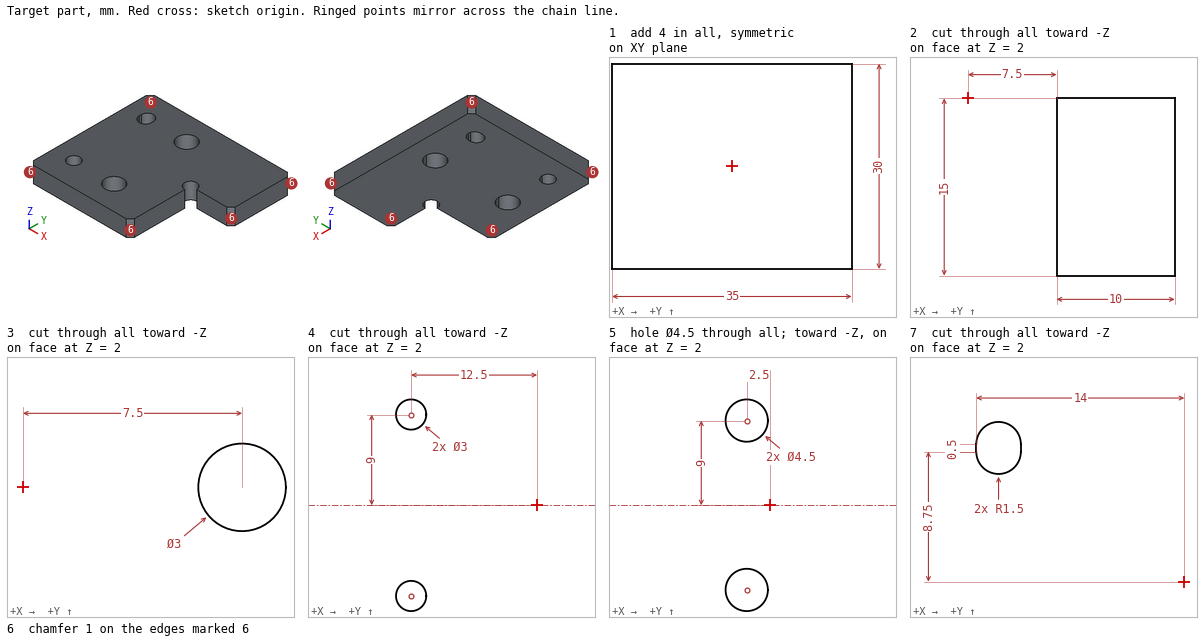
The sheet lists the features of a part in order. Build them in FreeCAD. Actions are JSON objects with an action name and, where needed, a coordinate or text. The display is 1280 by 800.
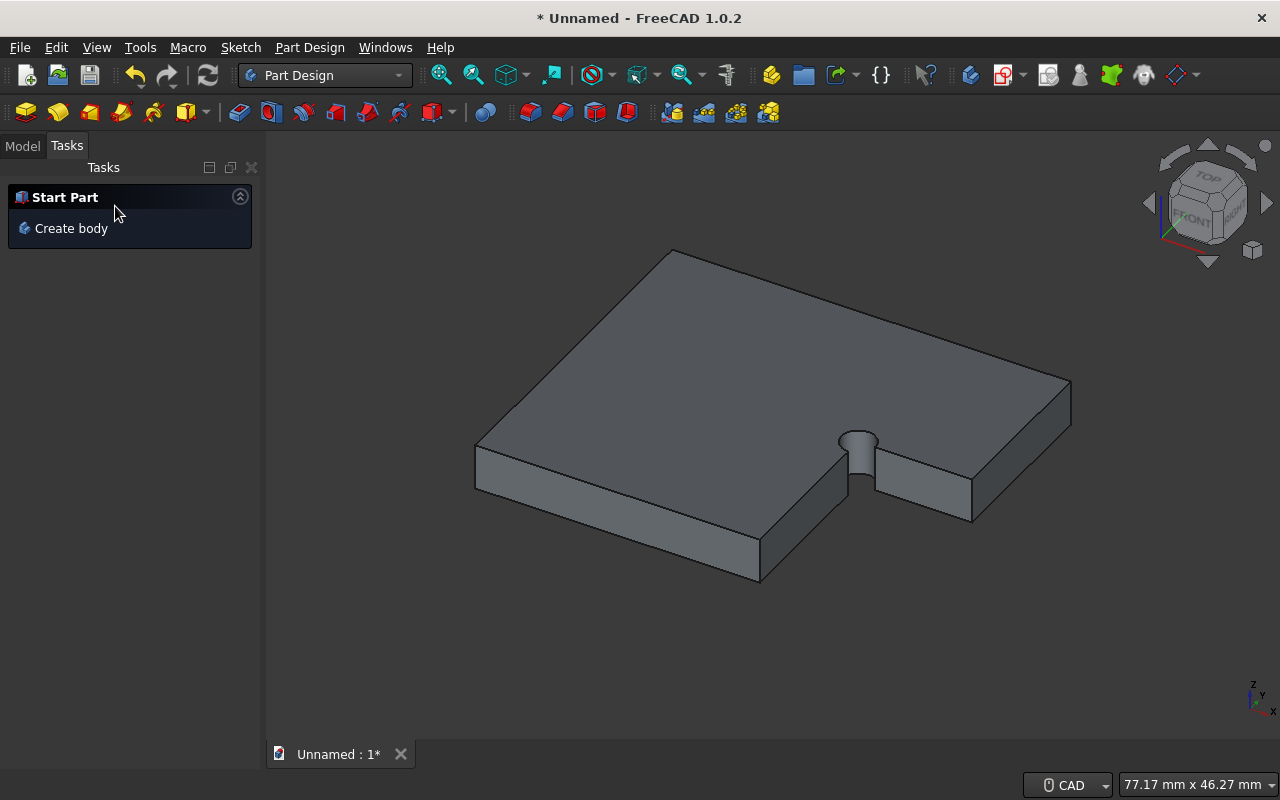
{"action": "left_click", "coordinate": [716, 394]}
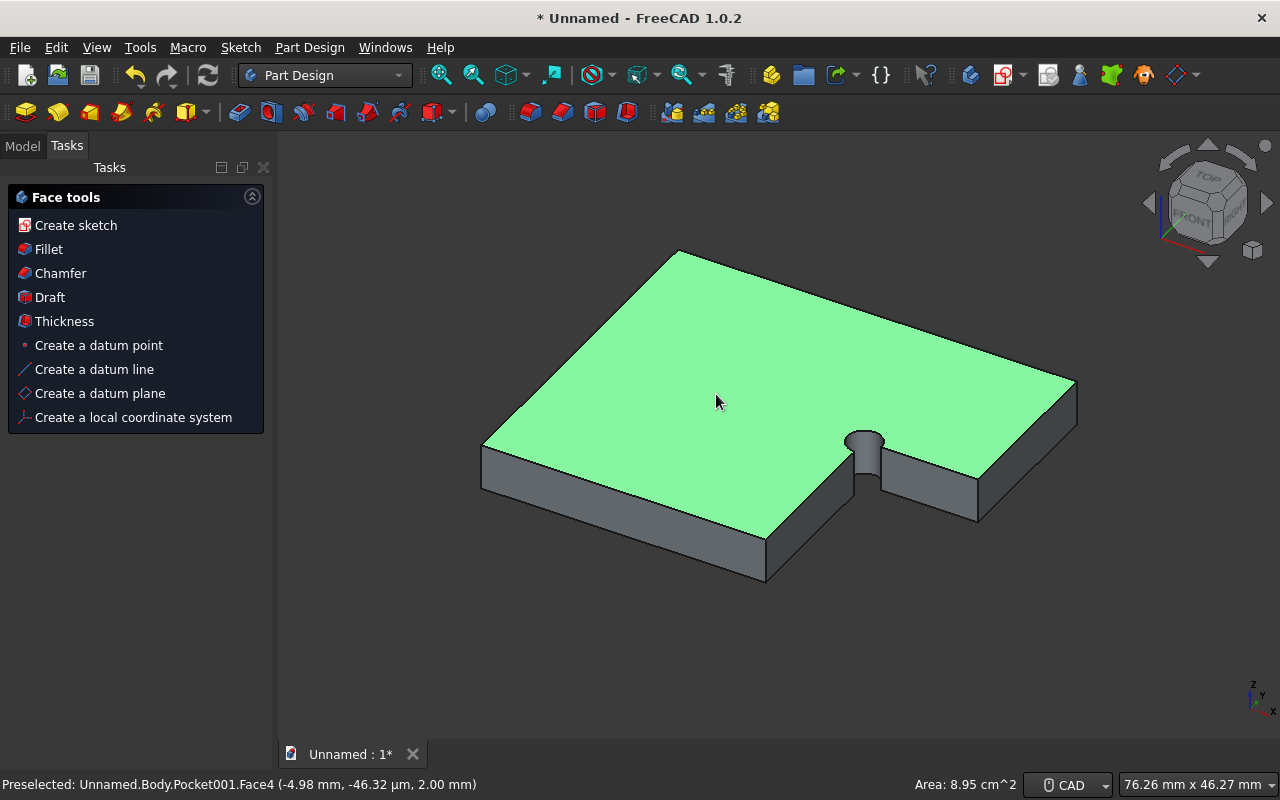
{"action": "left_click", "coordinate": [1004, 76]}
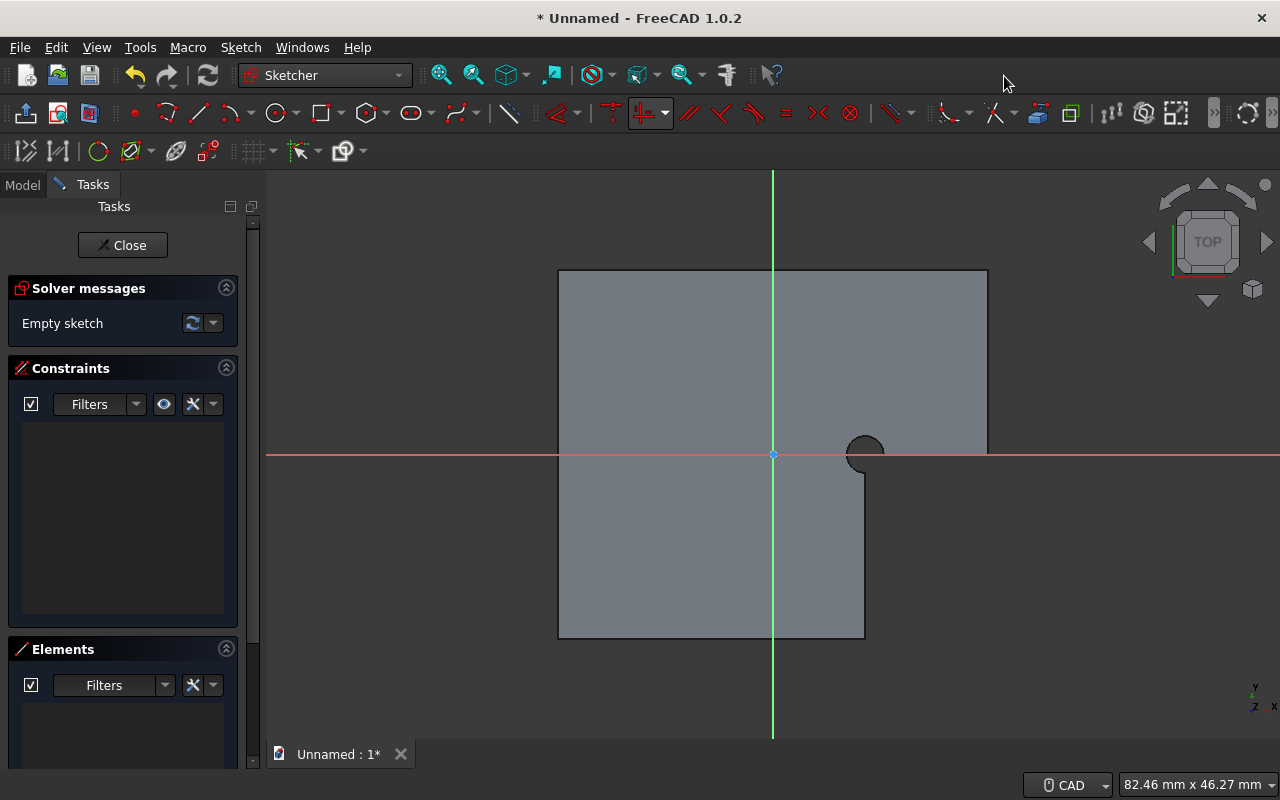
{"action": "scroll", "coordinate": [651, 455], "scroll_direction": "up", "scroll_amount": 2}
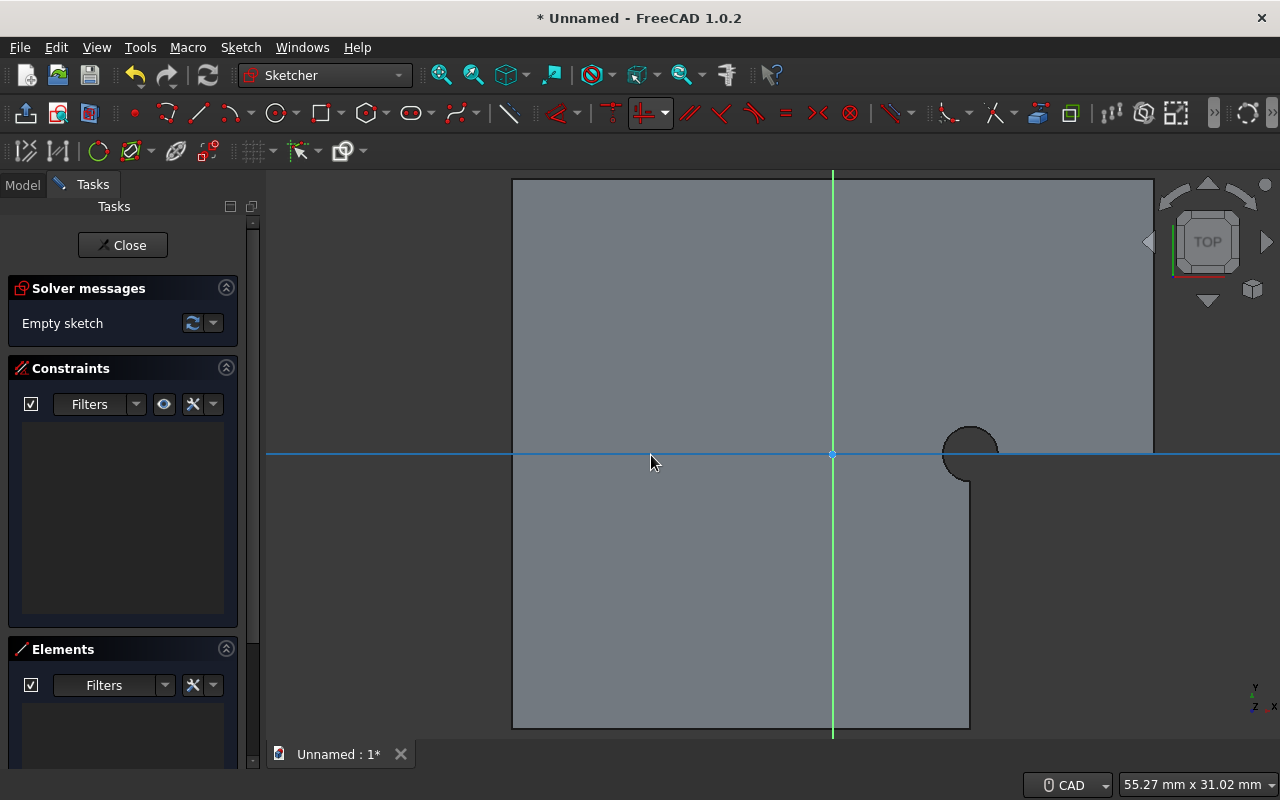
{"action": "key", "text": "g c"}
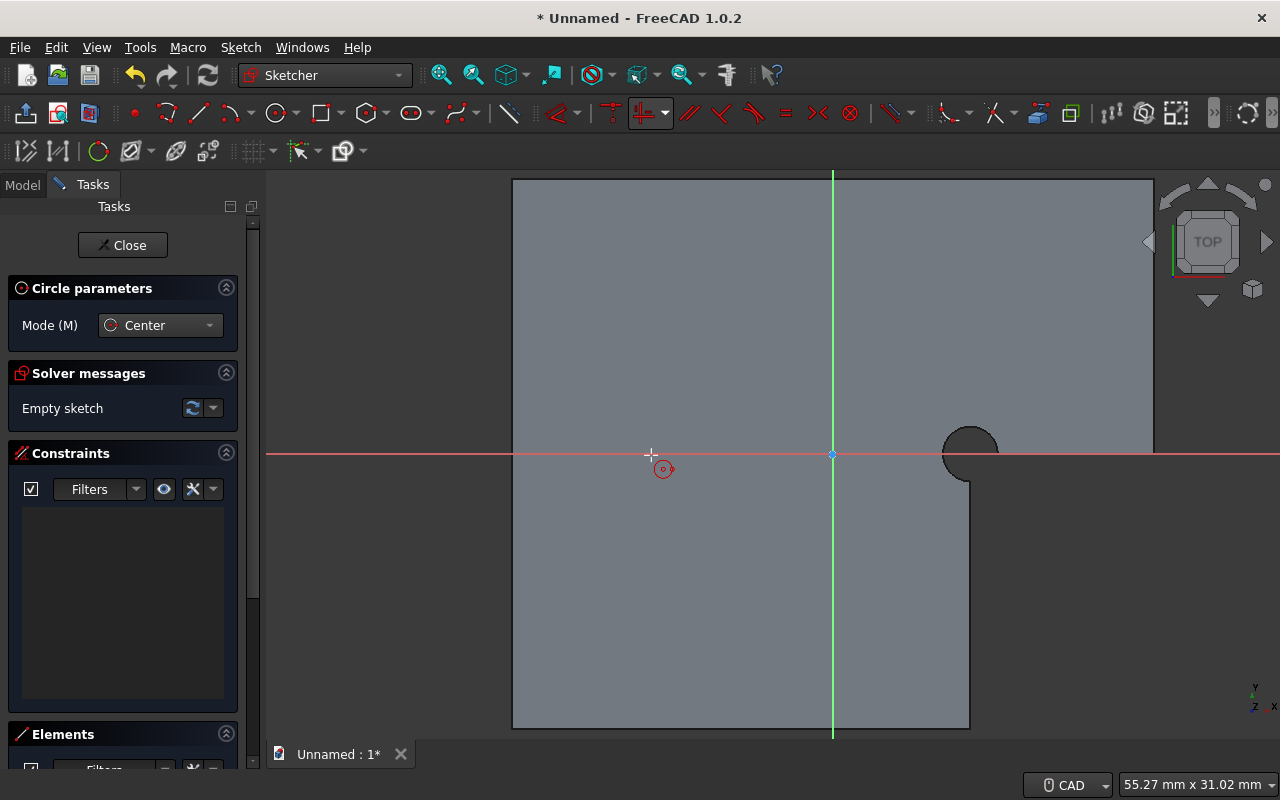
{"action": "left_click", "coordinate": [604, 289]}
{"action": "left_click", "coordinate": [623, 269]}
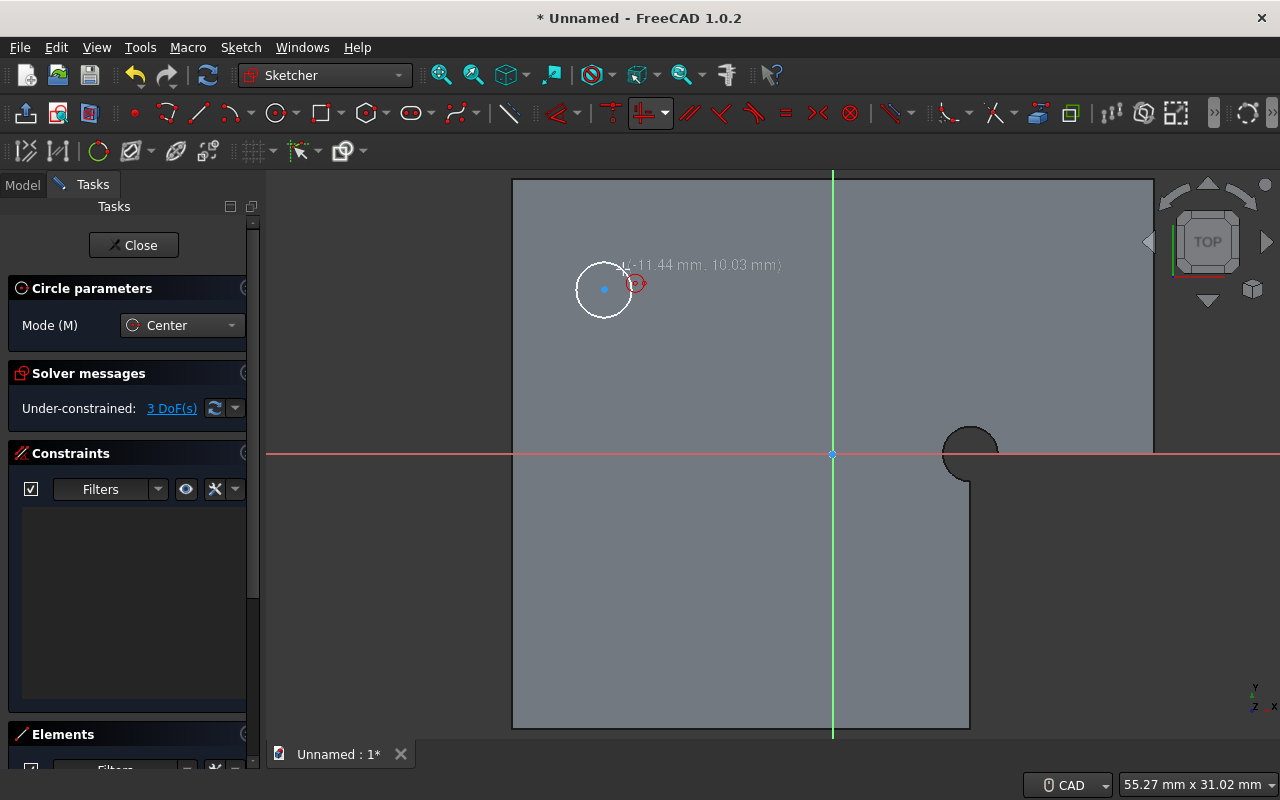
{"action": "left_click", "coordinate": [604, 619]}
{"action": "left_click", "coordinate": [623, 600]}
{"action": "key", "text": "Escape"}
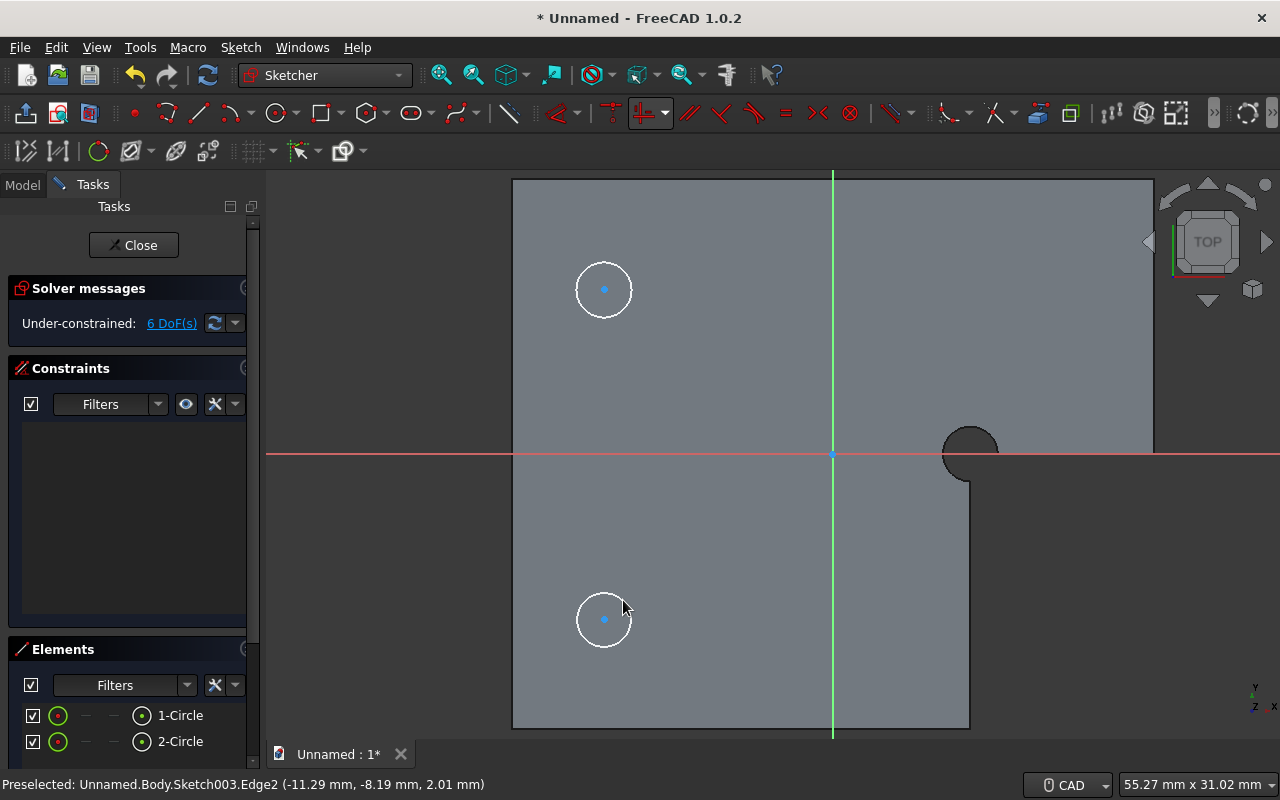
{"action": "left_click", "coordinate": [623, 270]}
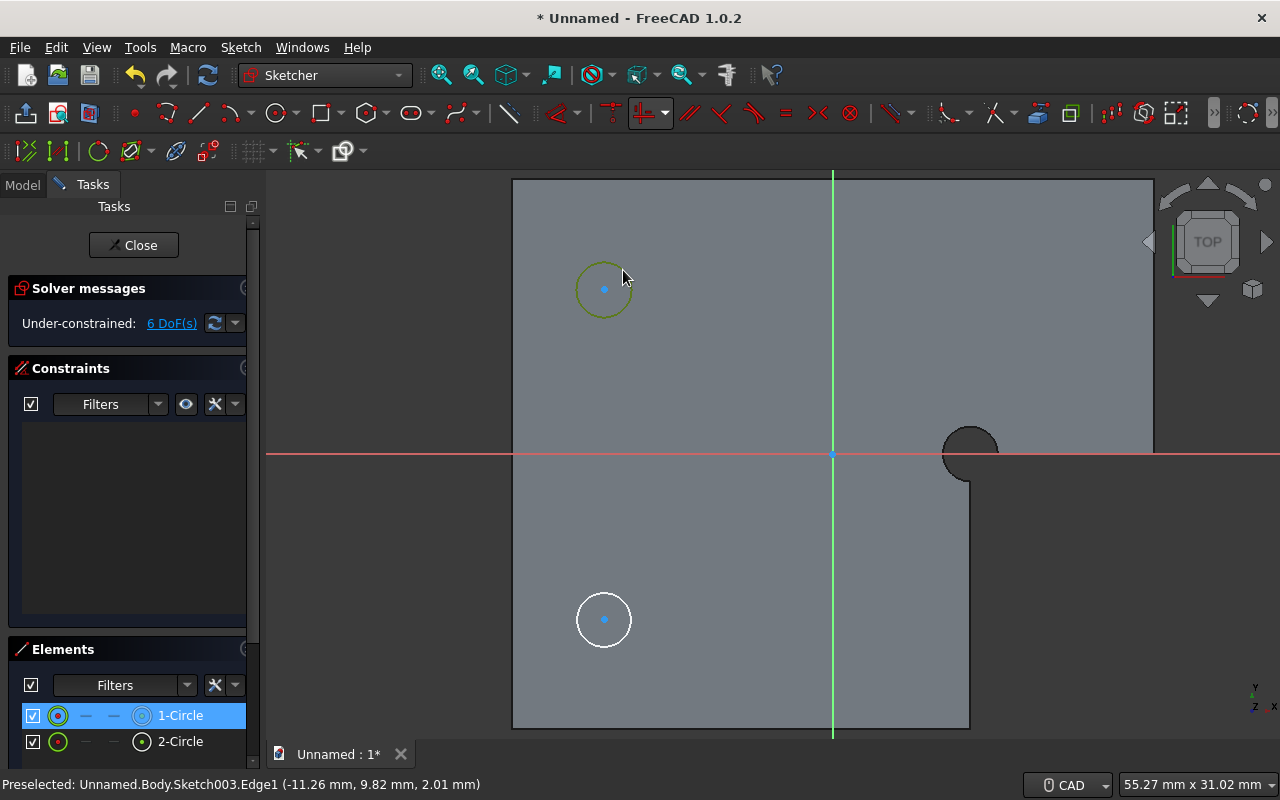
{"action": "left_click", "coordinate": [623, 601]}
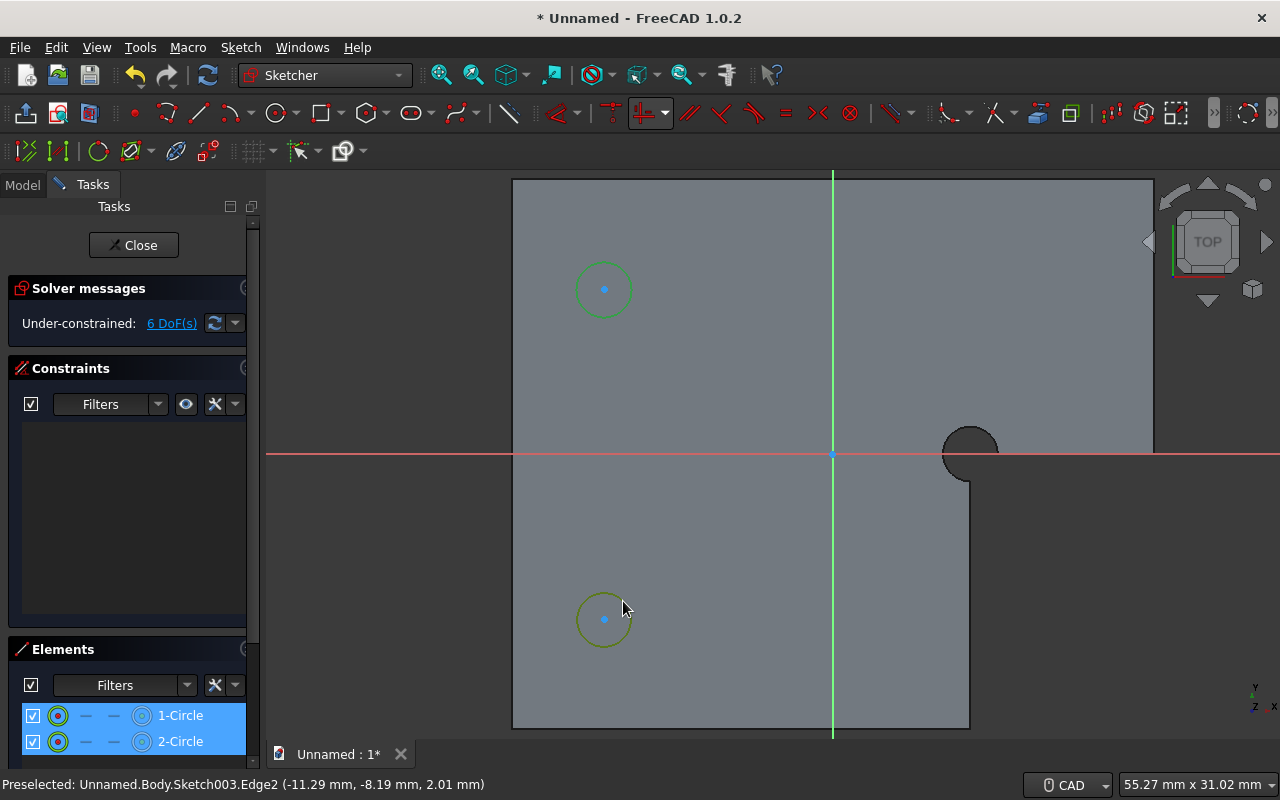
{"action": "key", "text": "e"}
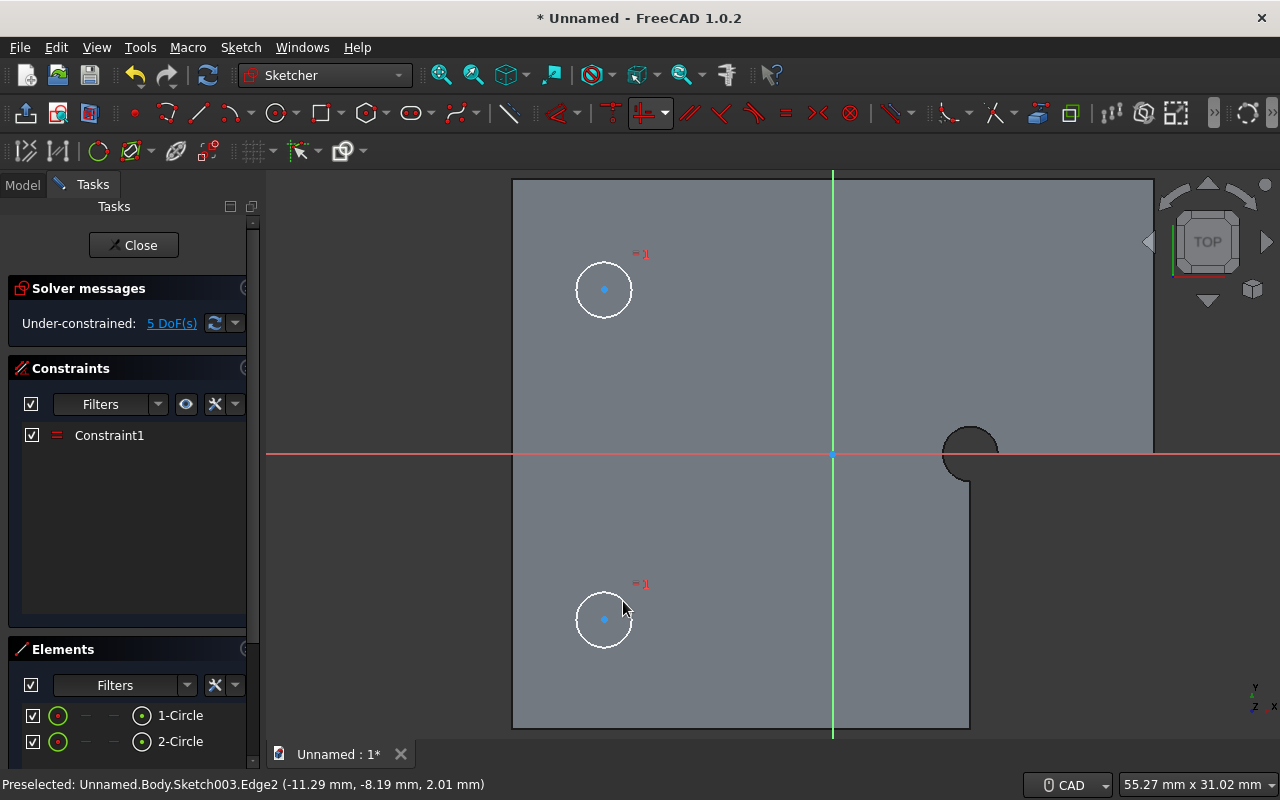
{"action": "left_click", "coordinate": [604, 290]}